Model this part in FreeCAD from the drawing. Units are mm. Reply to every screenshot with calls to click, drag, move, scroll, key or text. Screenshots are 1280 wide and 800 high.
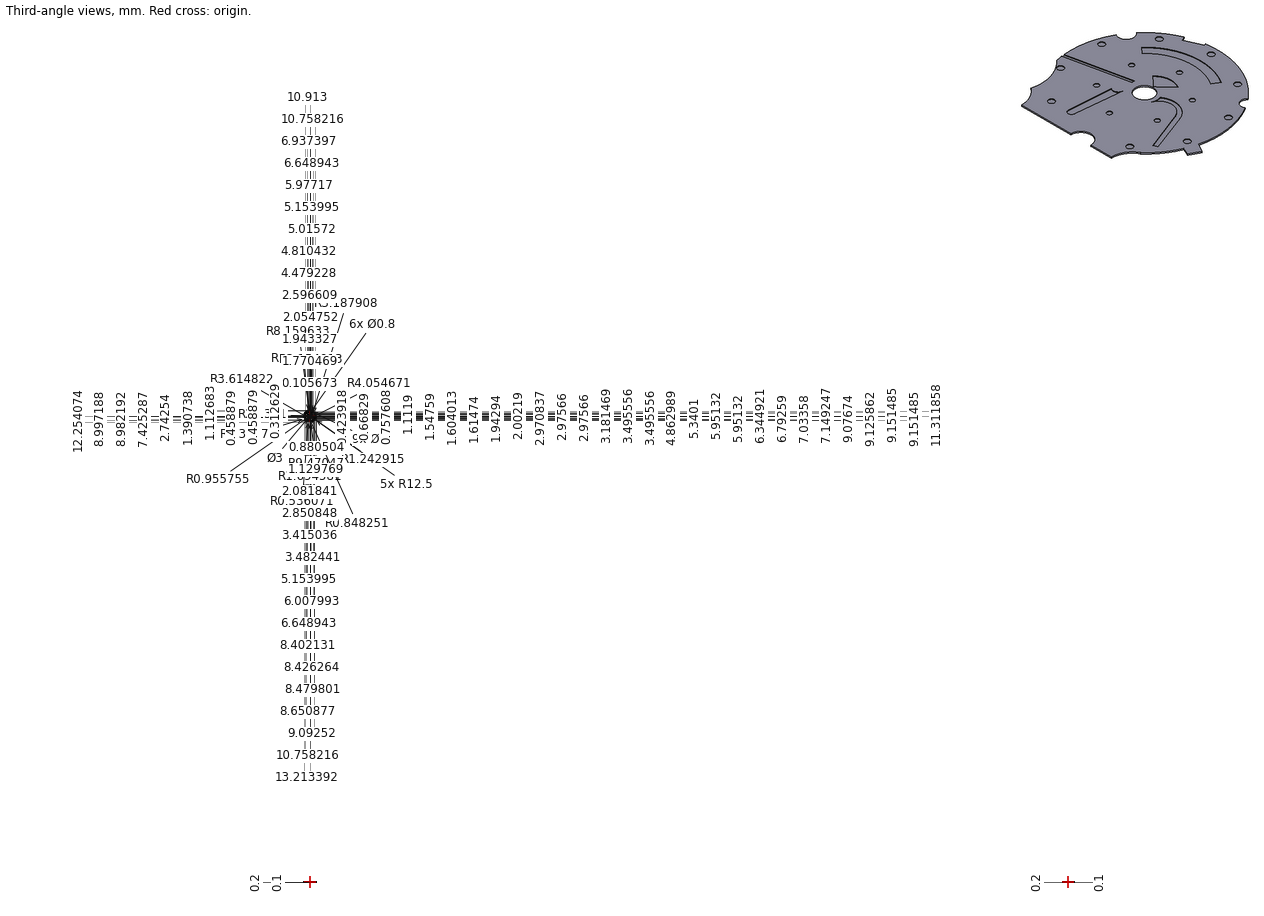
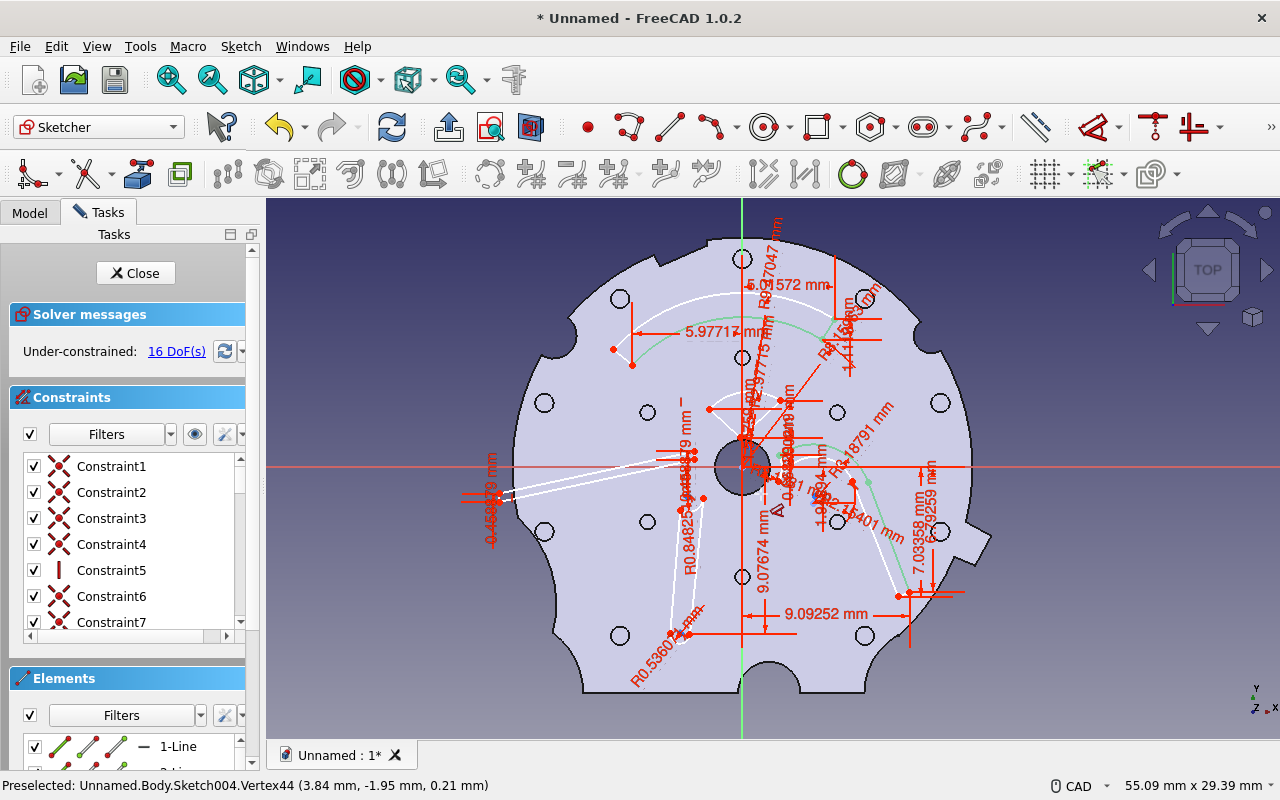
click(614, 350)
click(649, 501)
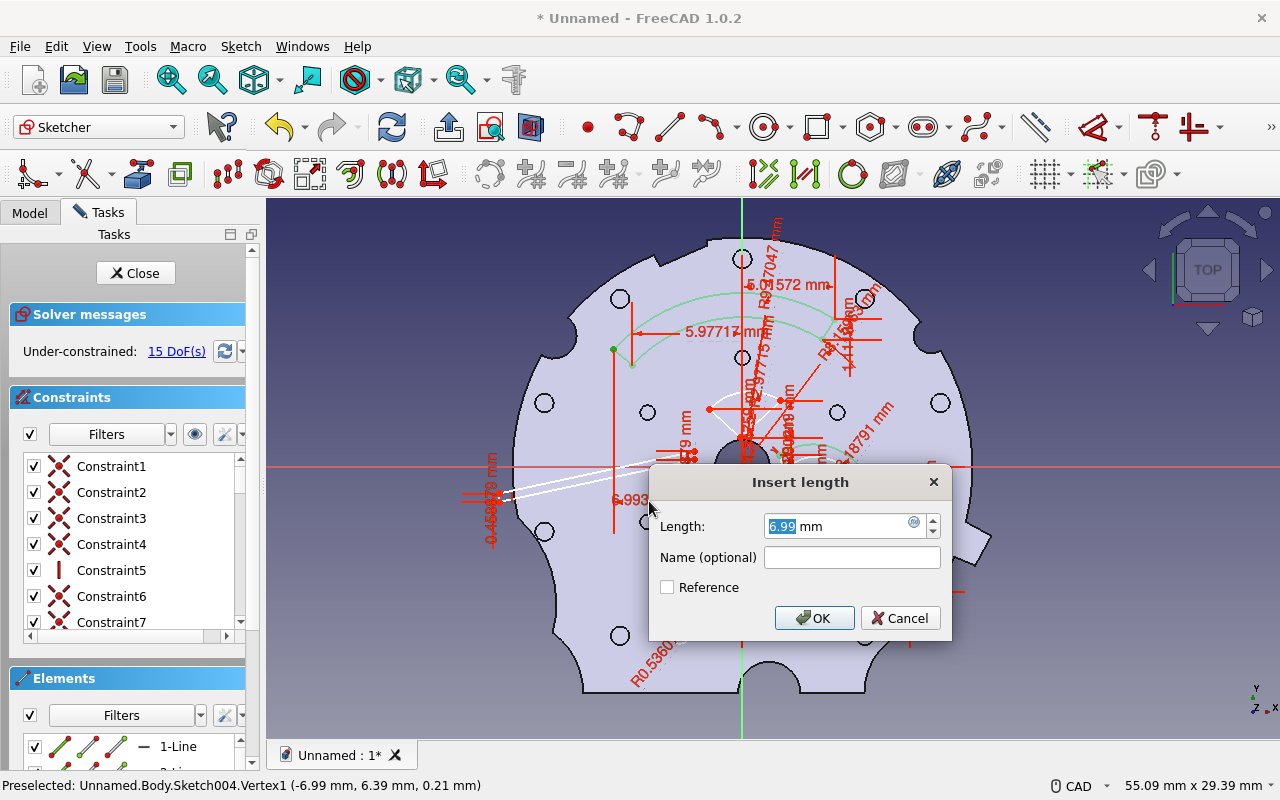
text(6.937397)
key(Return)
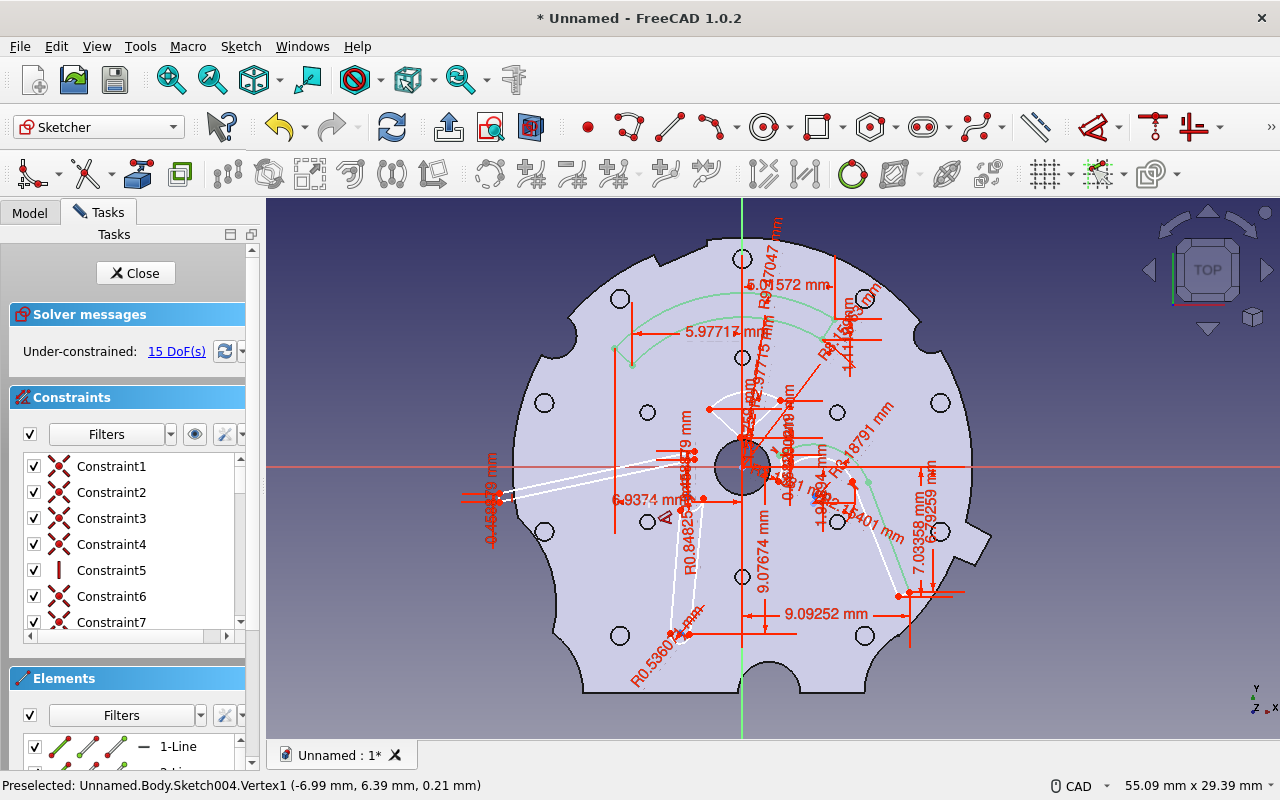
scroll(695, 460, up, 2)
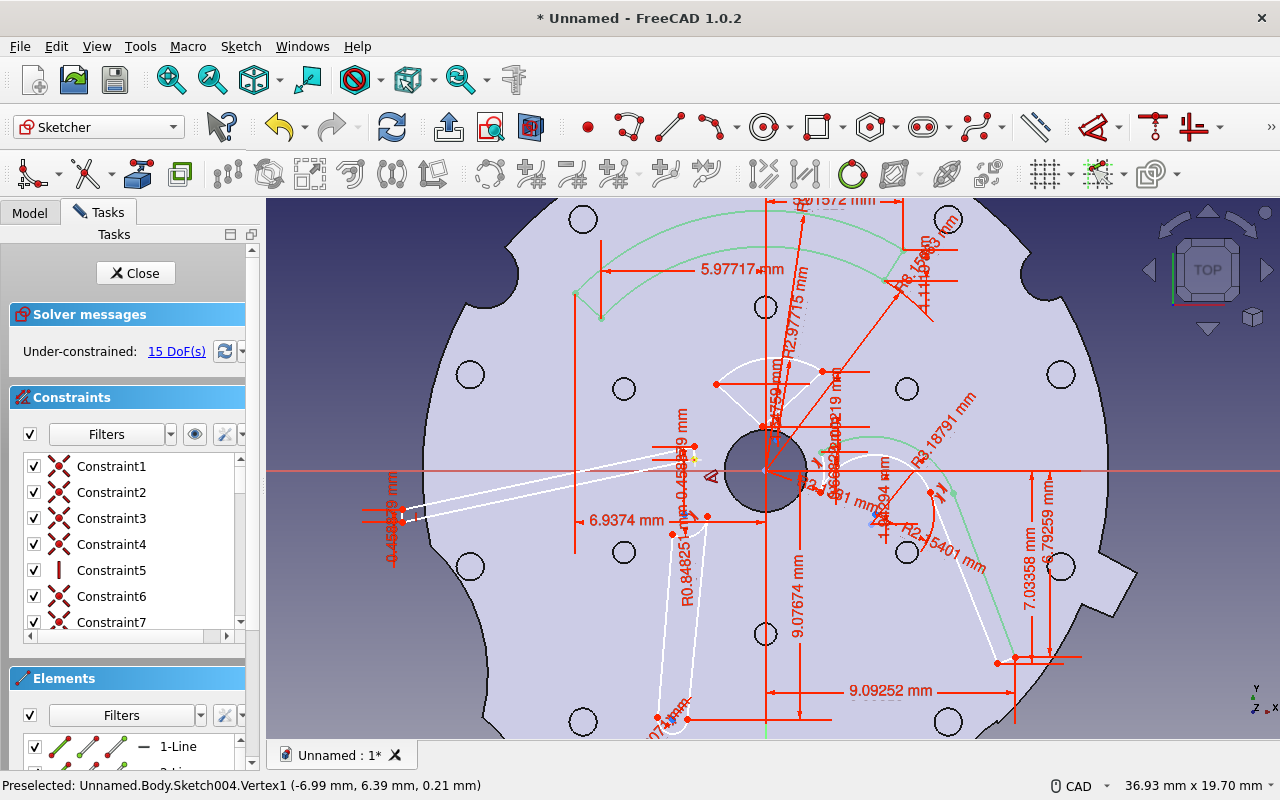
click(694, 460)
click(730, 426)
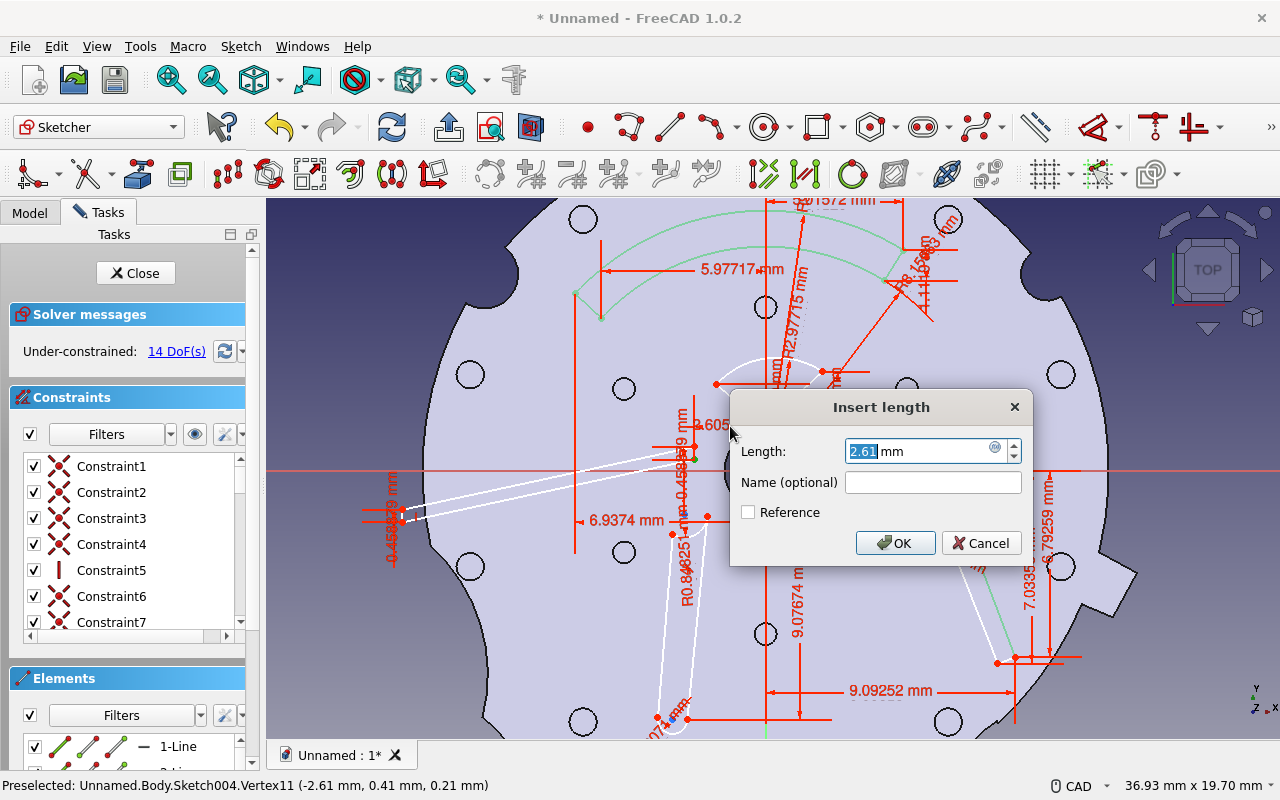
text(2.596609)
key(Return)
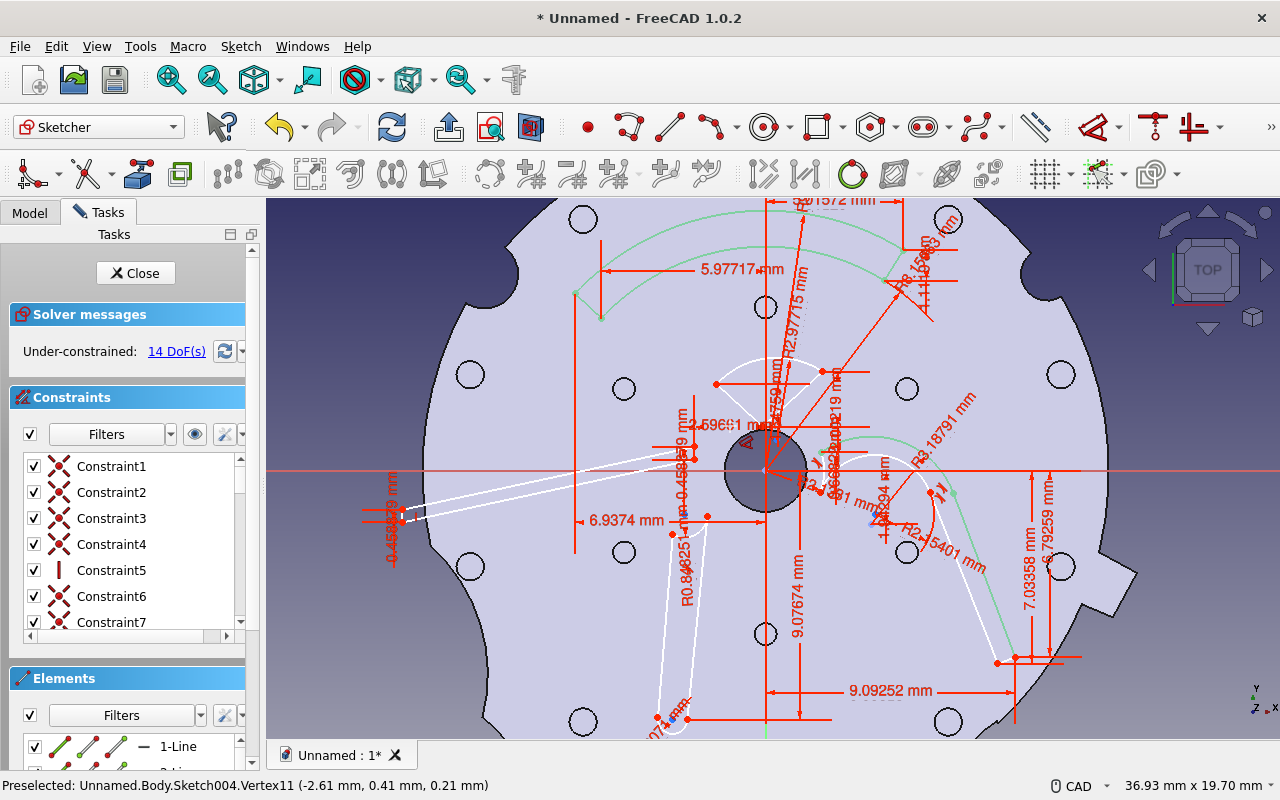
scroll(694, 460, up, 7)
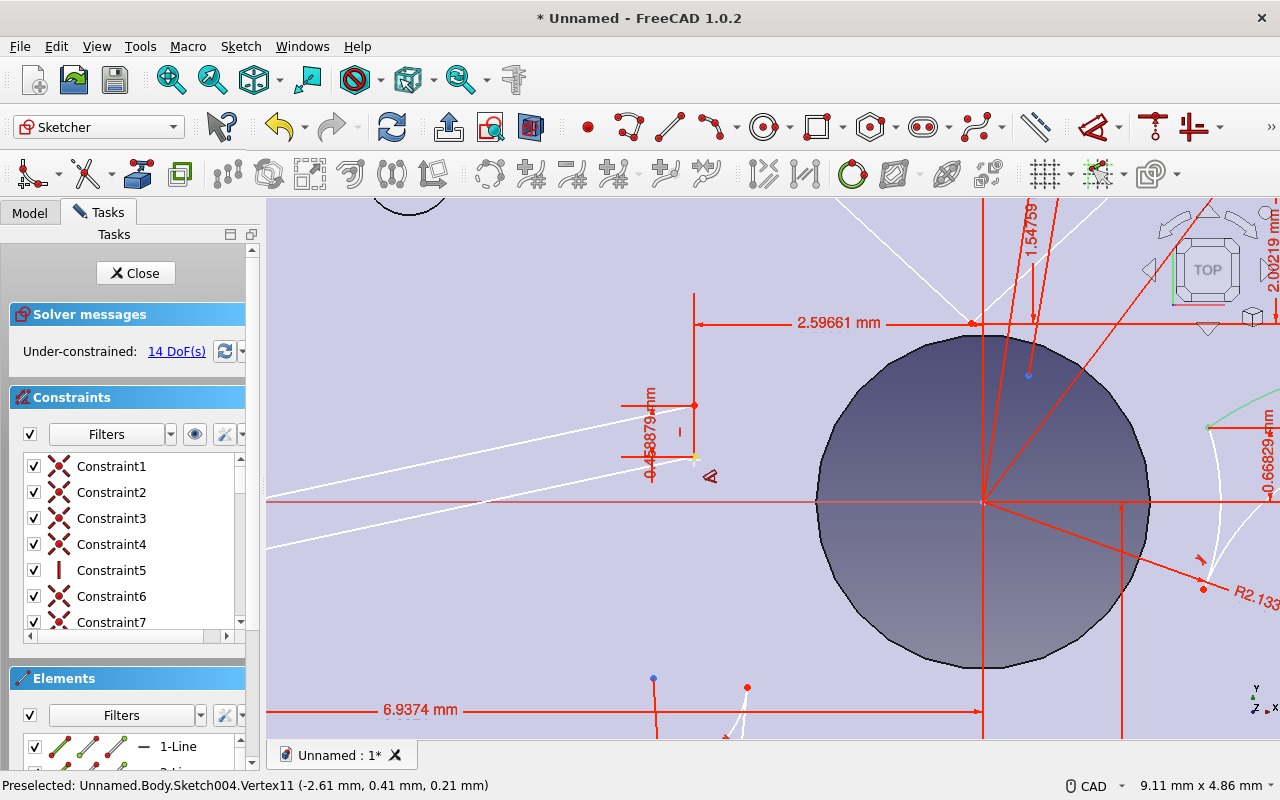
click(694, 457)
click(1017, 479)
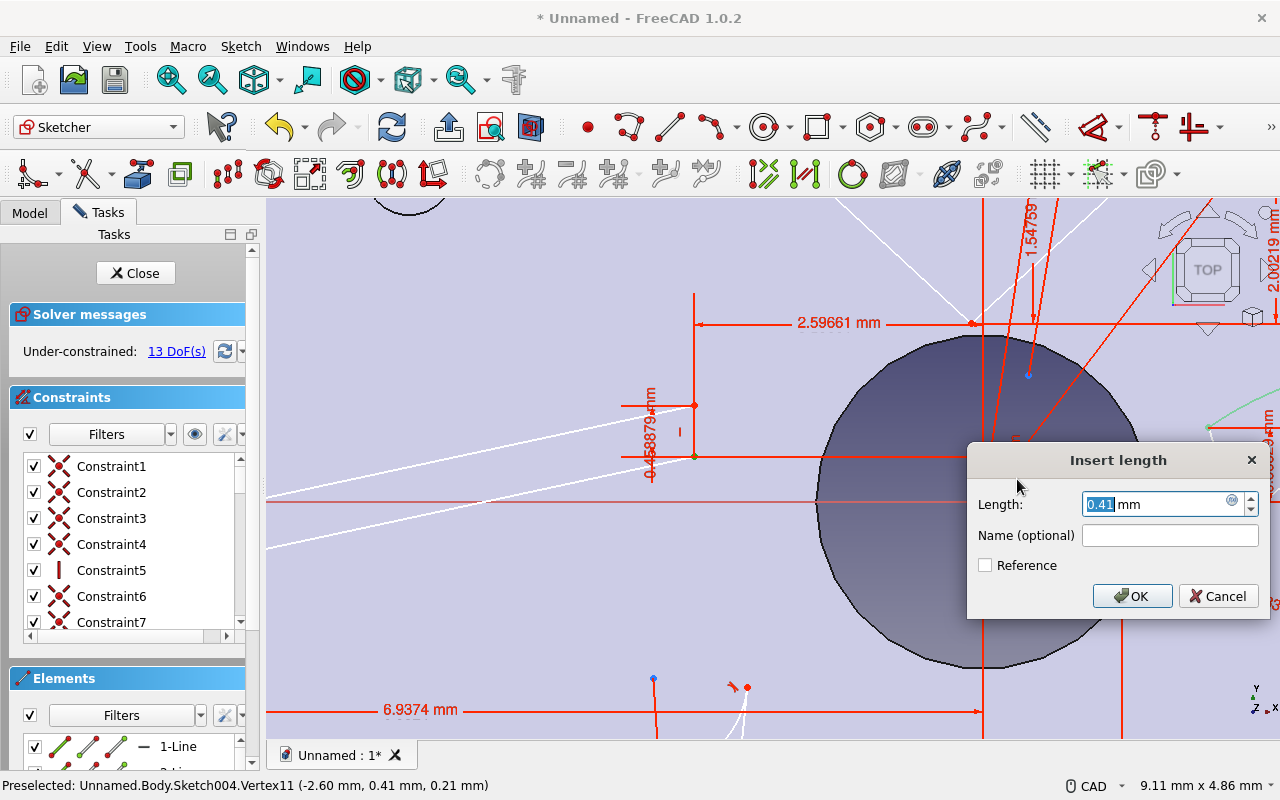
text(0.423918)
key(Return)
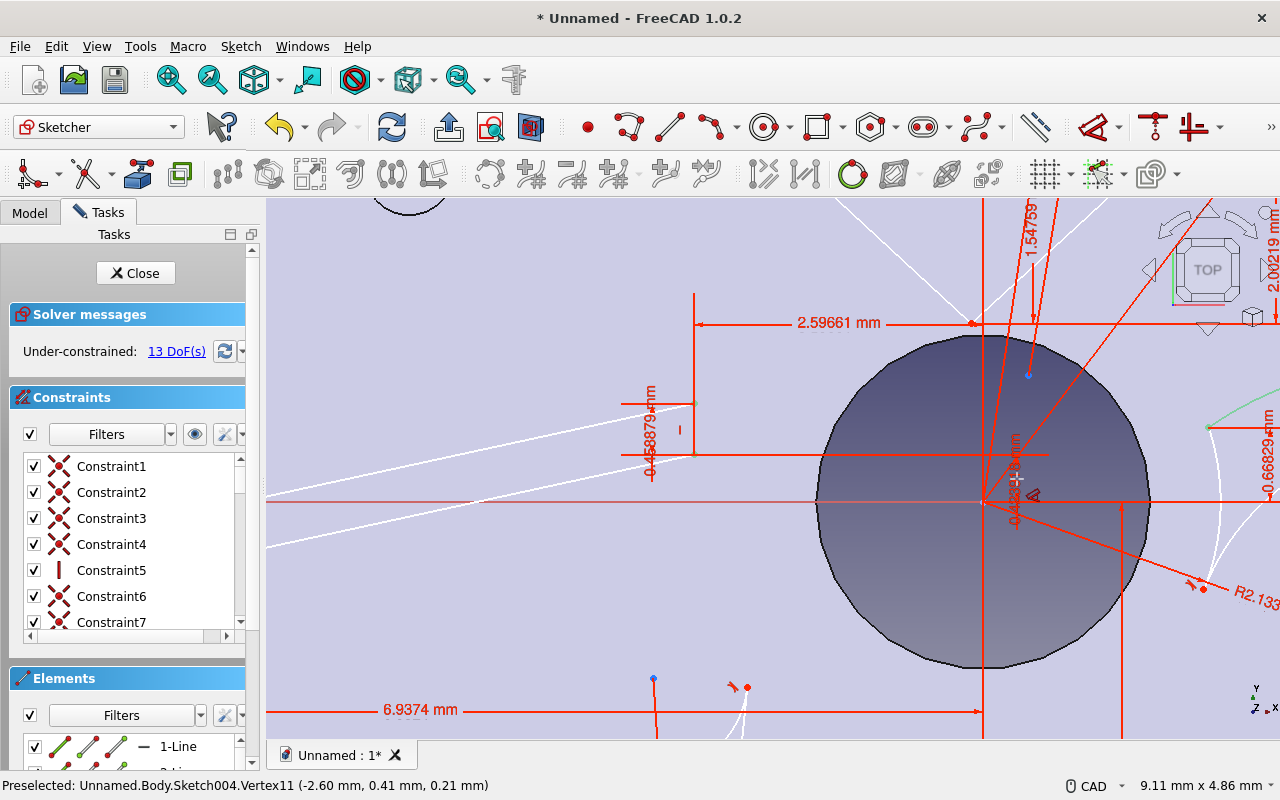
scroll(695, 460, down, 9)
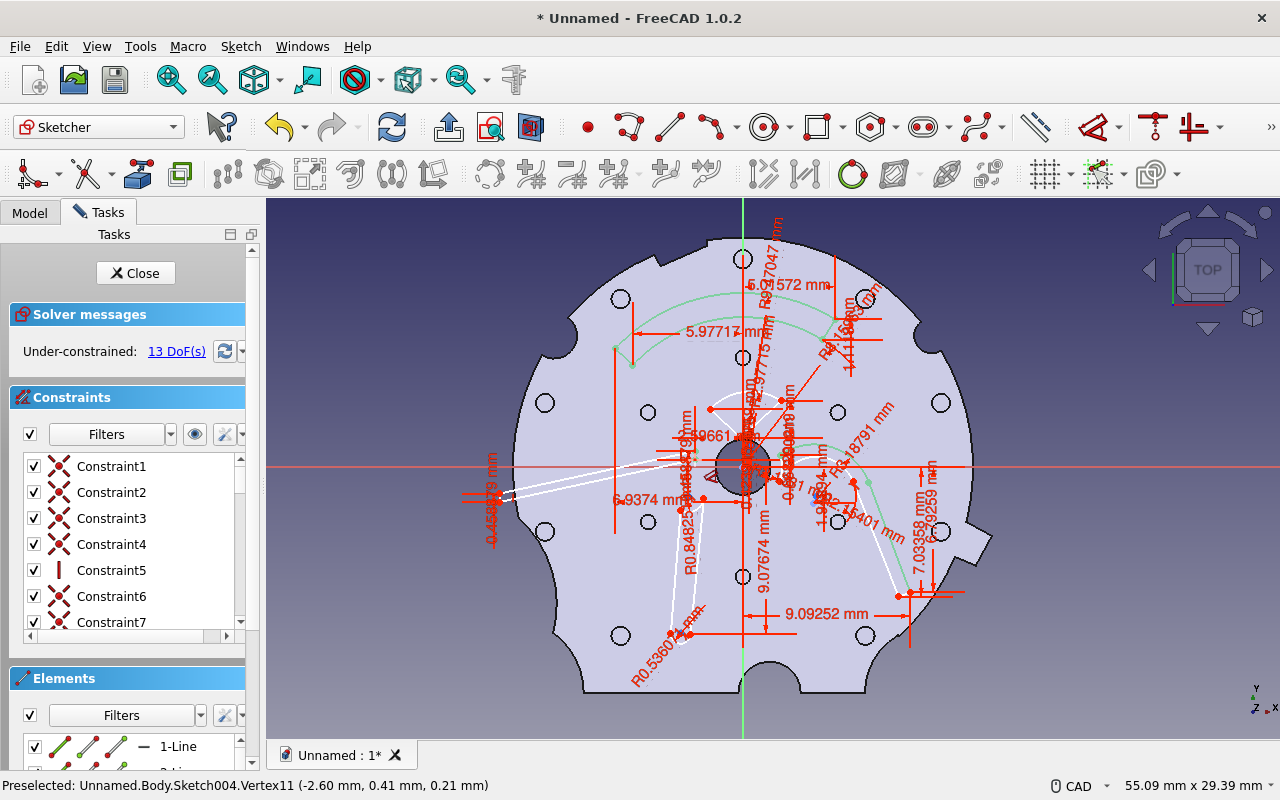
scroll(500, 494, up, 3)